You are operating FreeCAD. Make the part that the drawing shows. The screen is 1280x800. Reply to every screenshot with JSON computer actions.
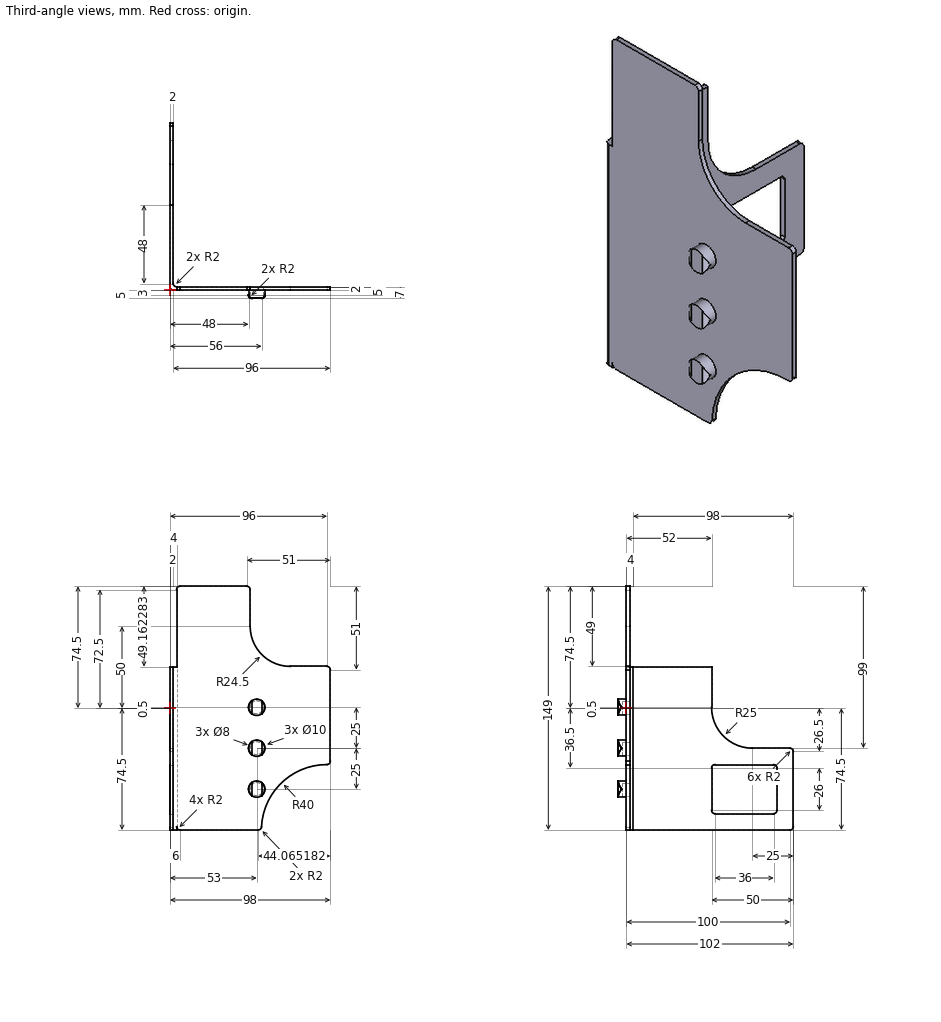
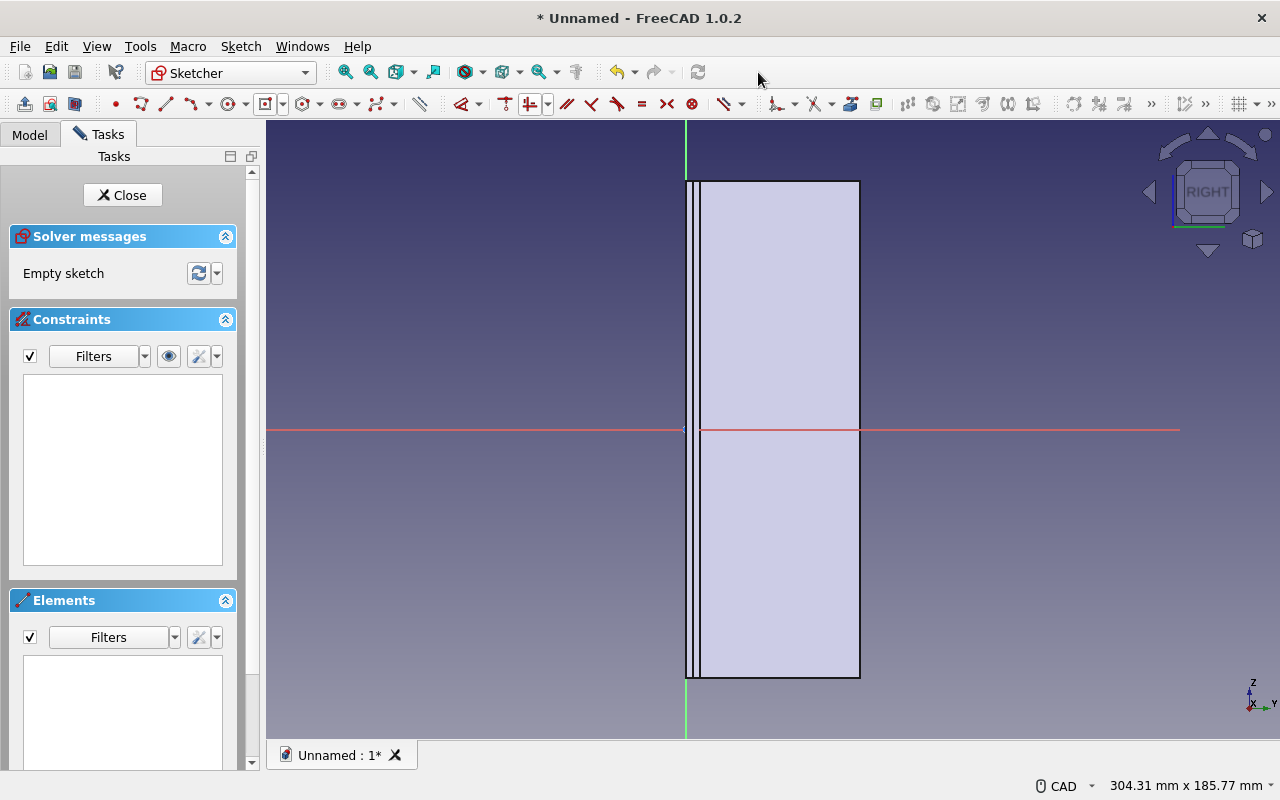
{"action": "key", "text": "q s"}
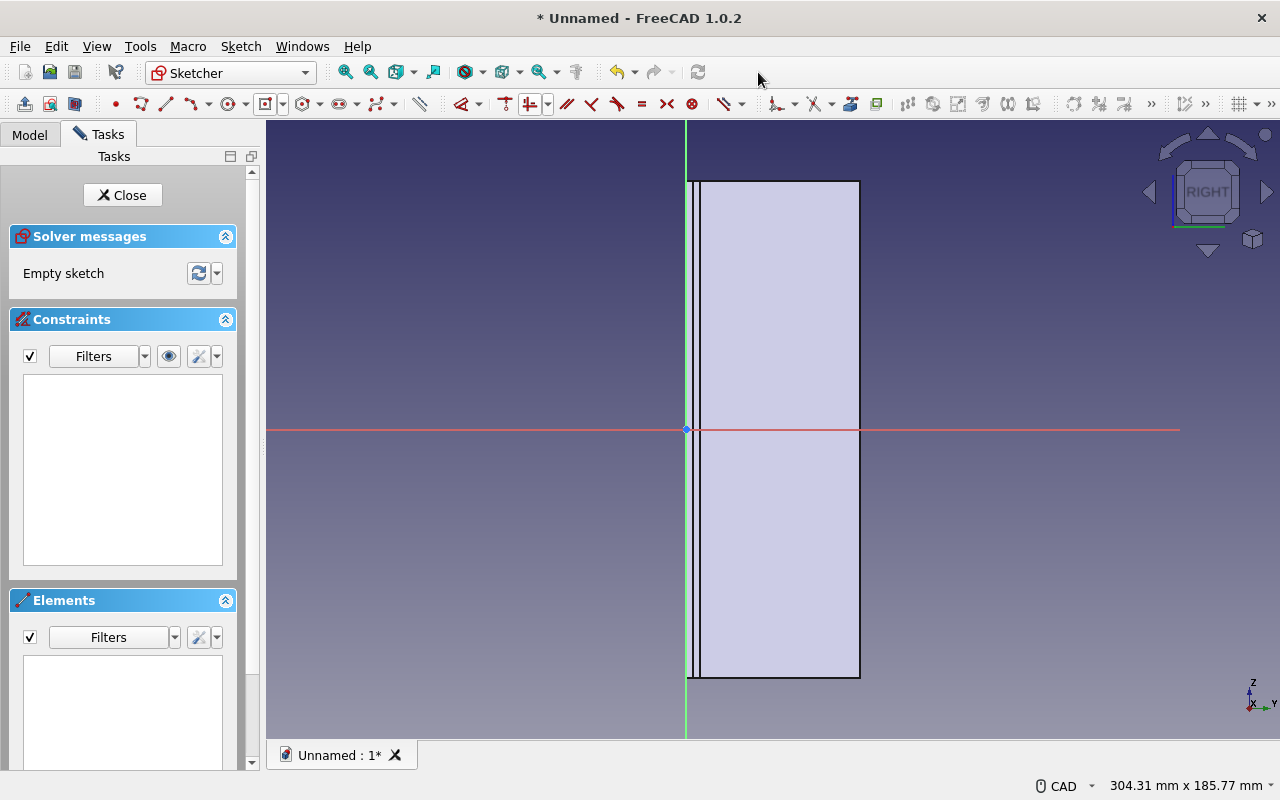
{"action": "left_click", "coordinate": [282, 104]}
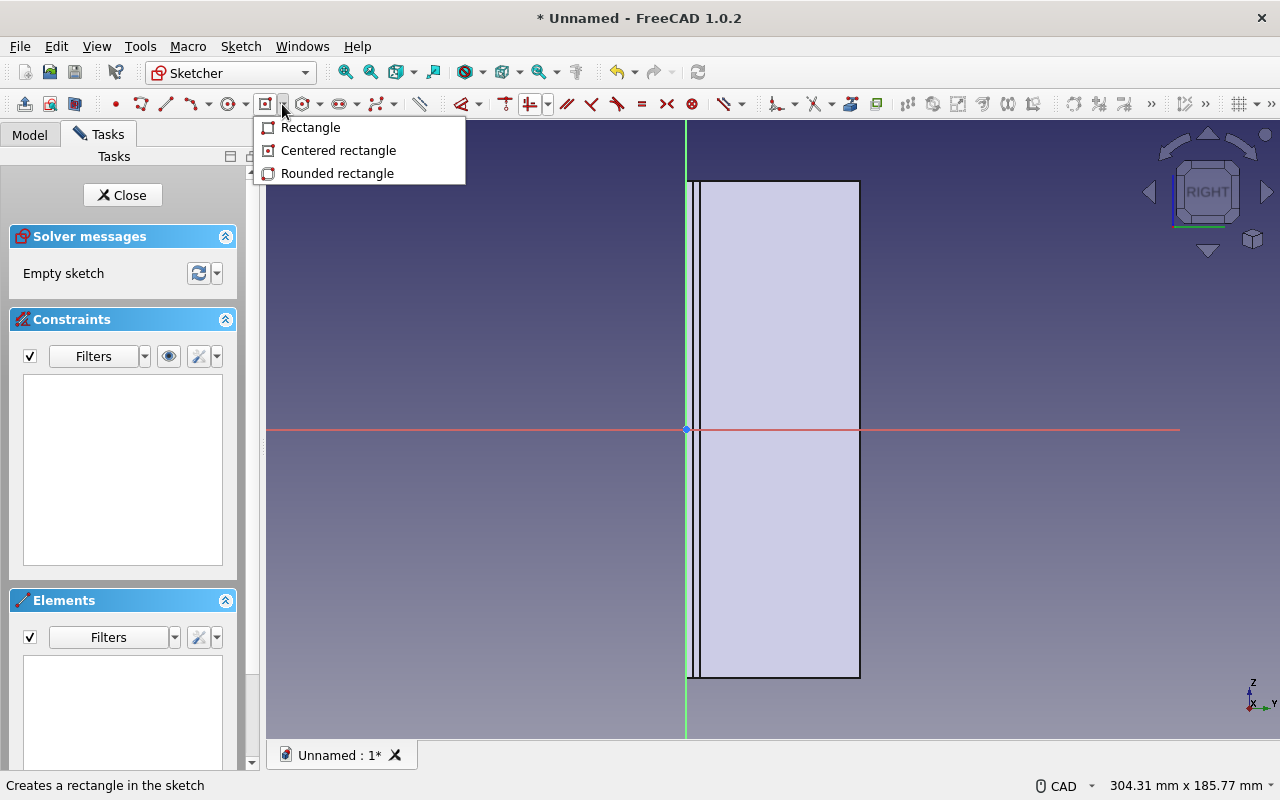
{"action": "left_click", "coordinate": [360, 128]}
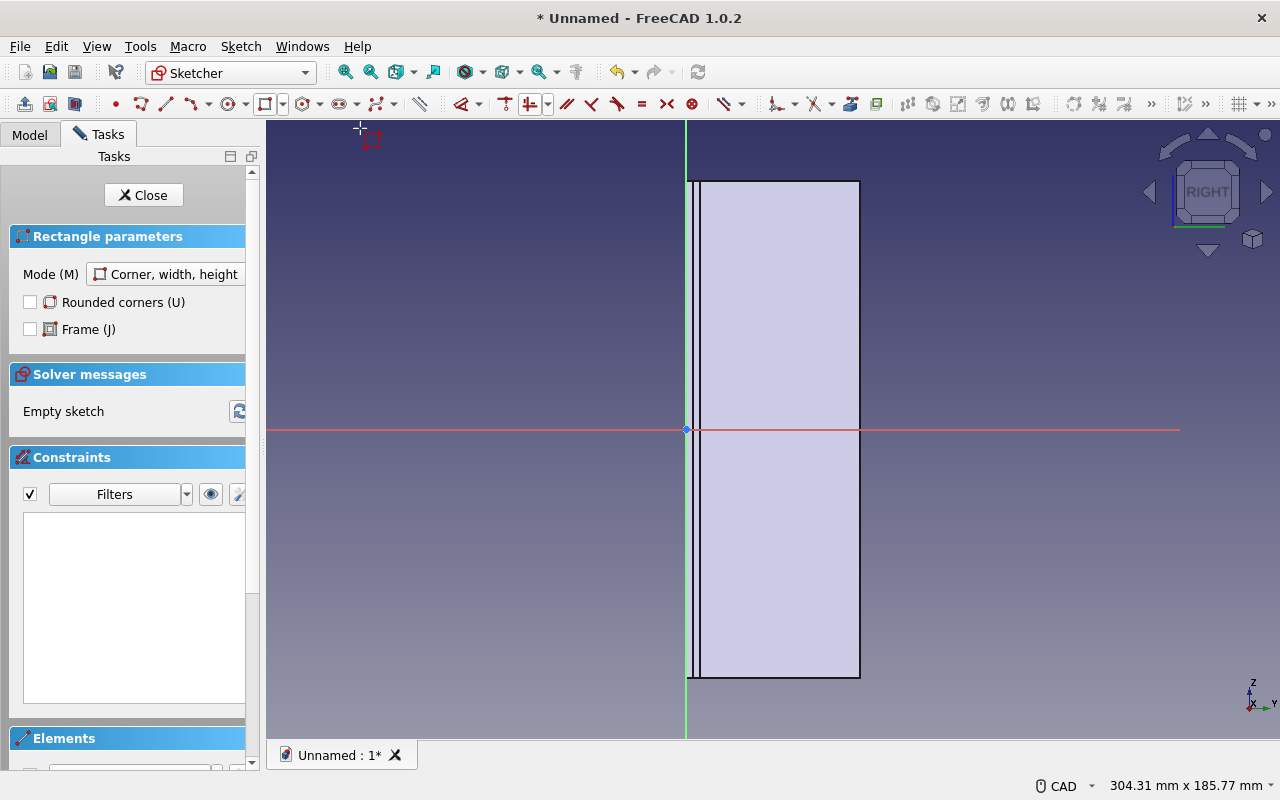
{"action": "left_click", "coordinate": [860, 181]}
{"action": "mouse_move", "coordinate": [1026, 678]}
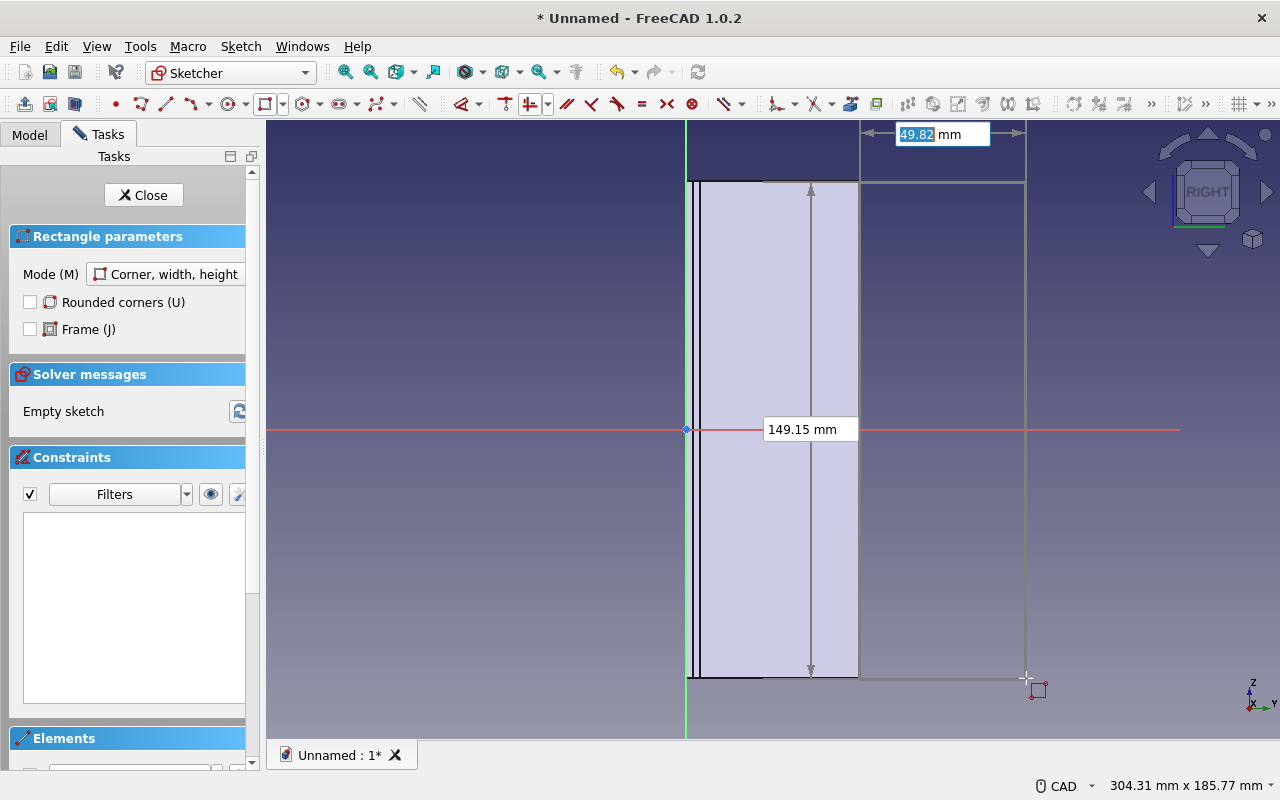
{"action": "type", "text": "50"}
{"action": "key", "text": "Tab"}
{"action": "type", "text": "149"}
{"action": "key", "text": "Return"}
{"action": "key", "text": "Escape"}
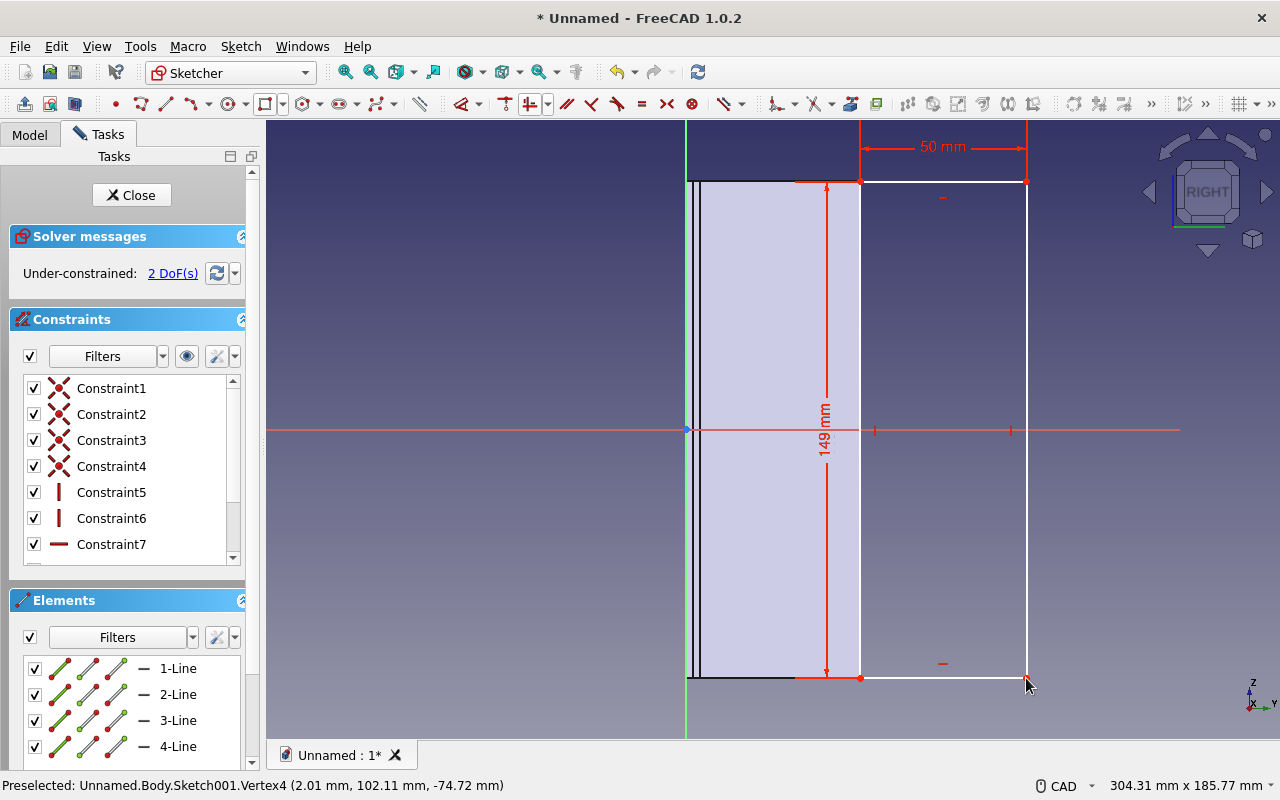
{"action": "left_click", "coordinate": [860, 182]}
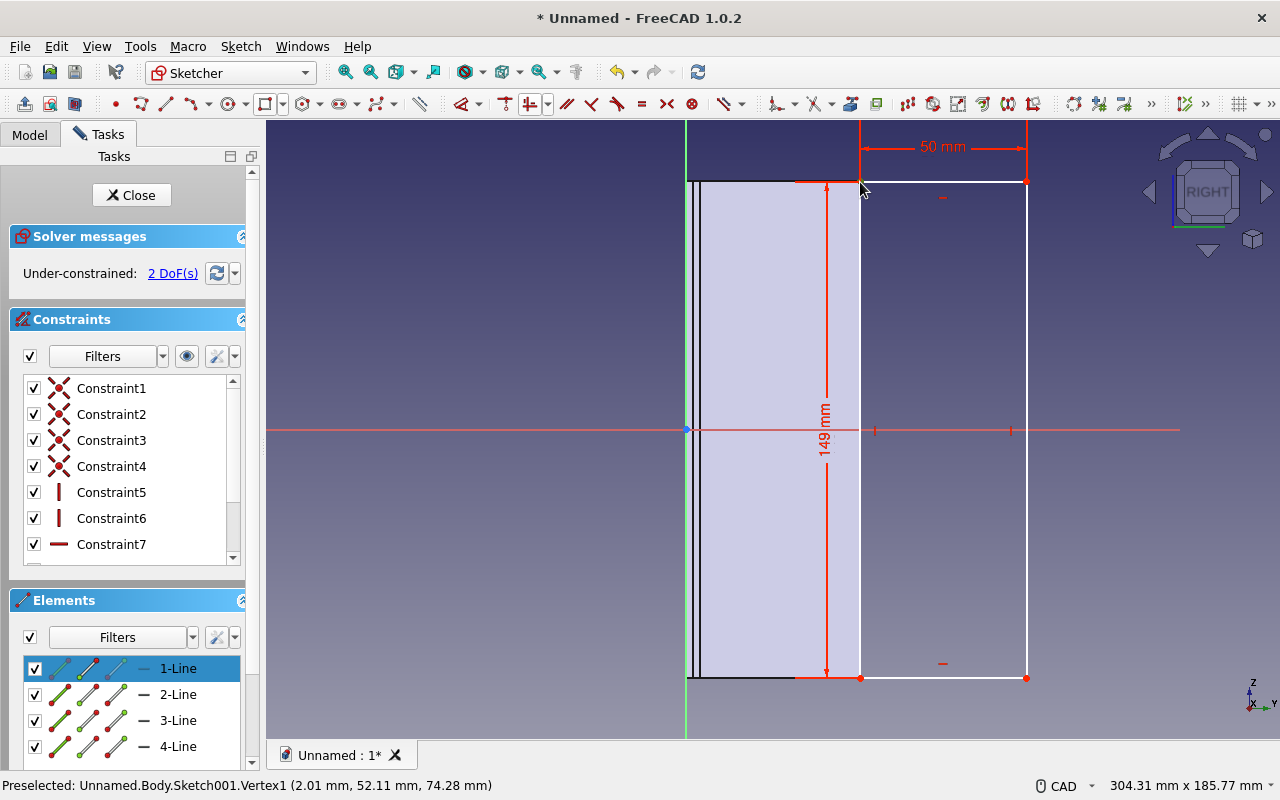
{"action": "key", "text": "l"}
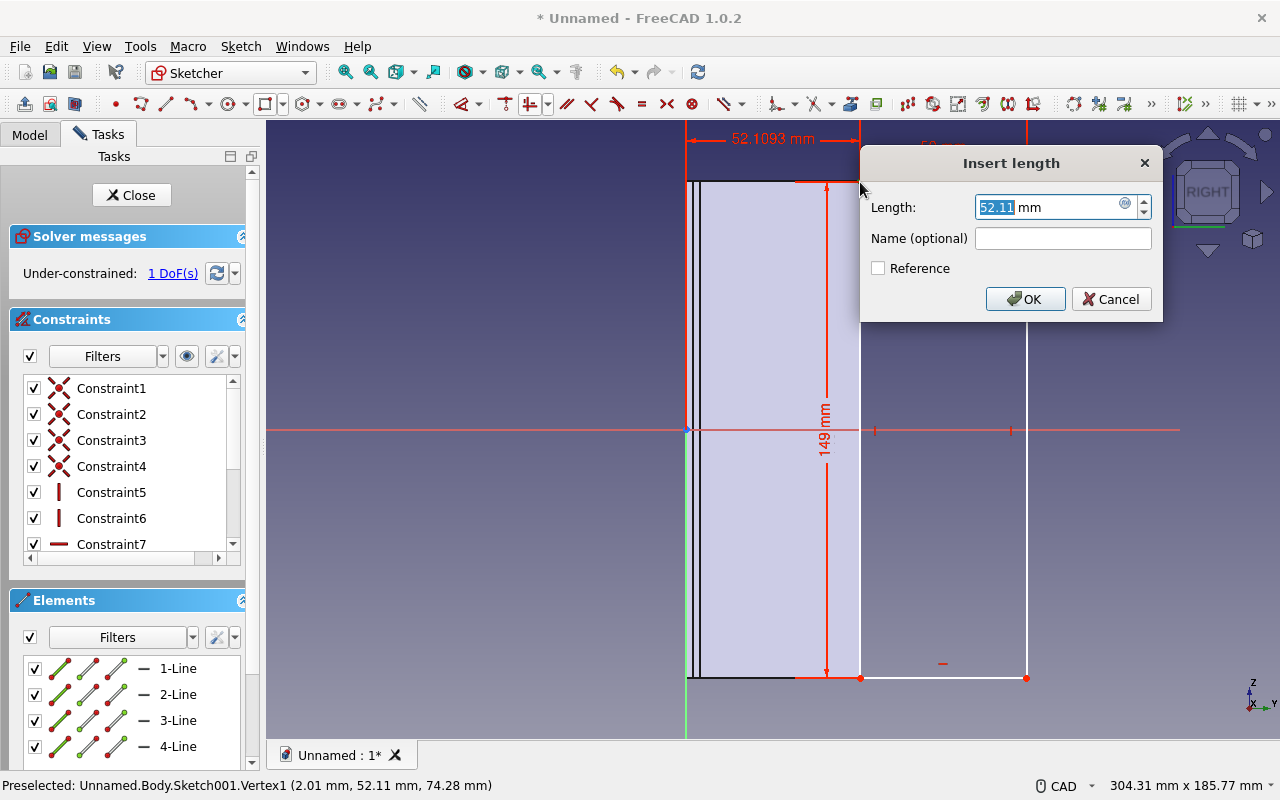
{"action": "type", "text": "52"}
{"action": "key", "text": "Return"}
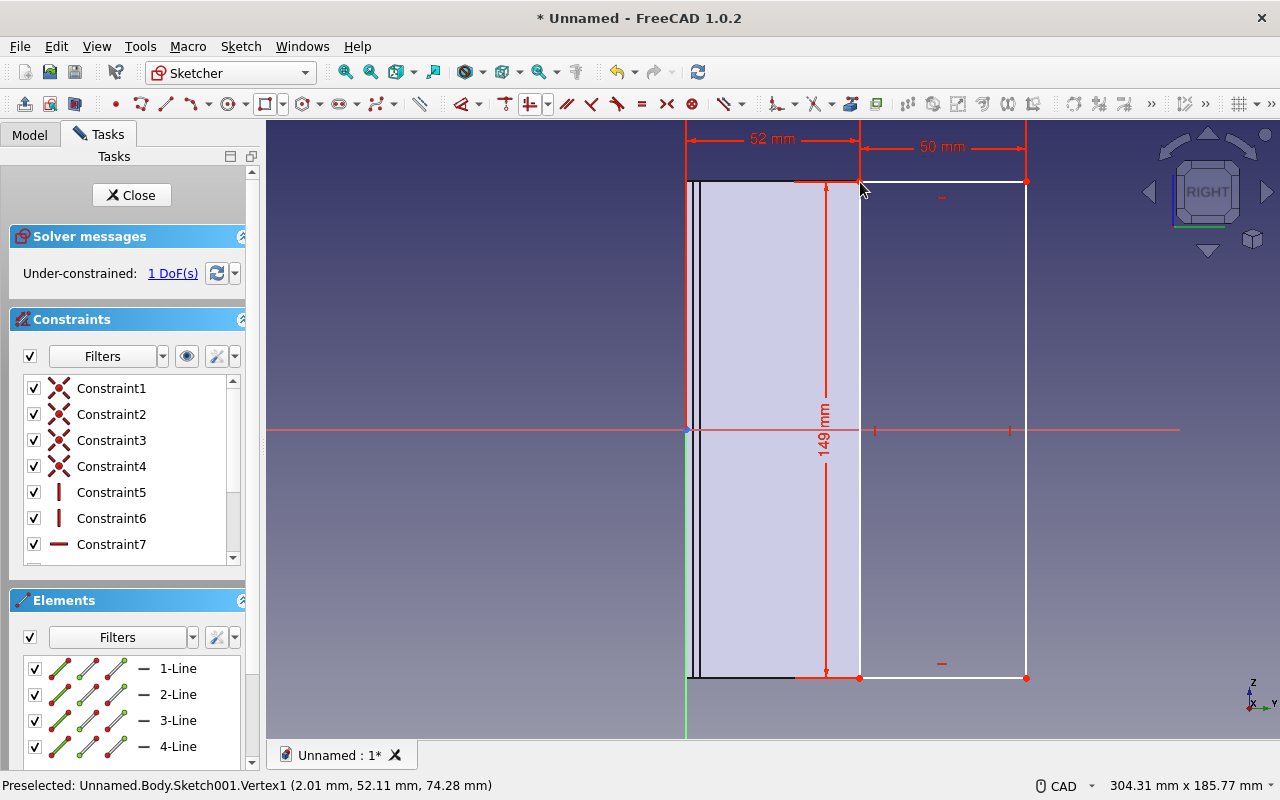
{"action": "left_click", "coordinate": [860, 182]}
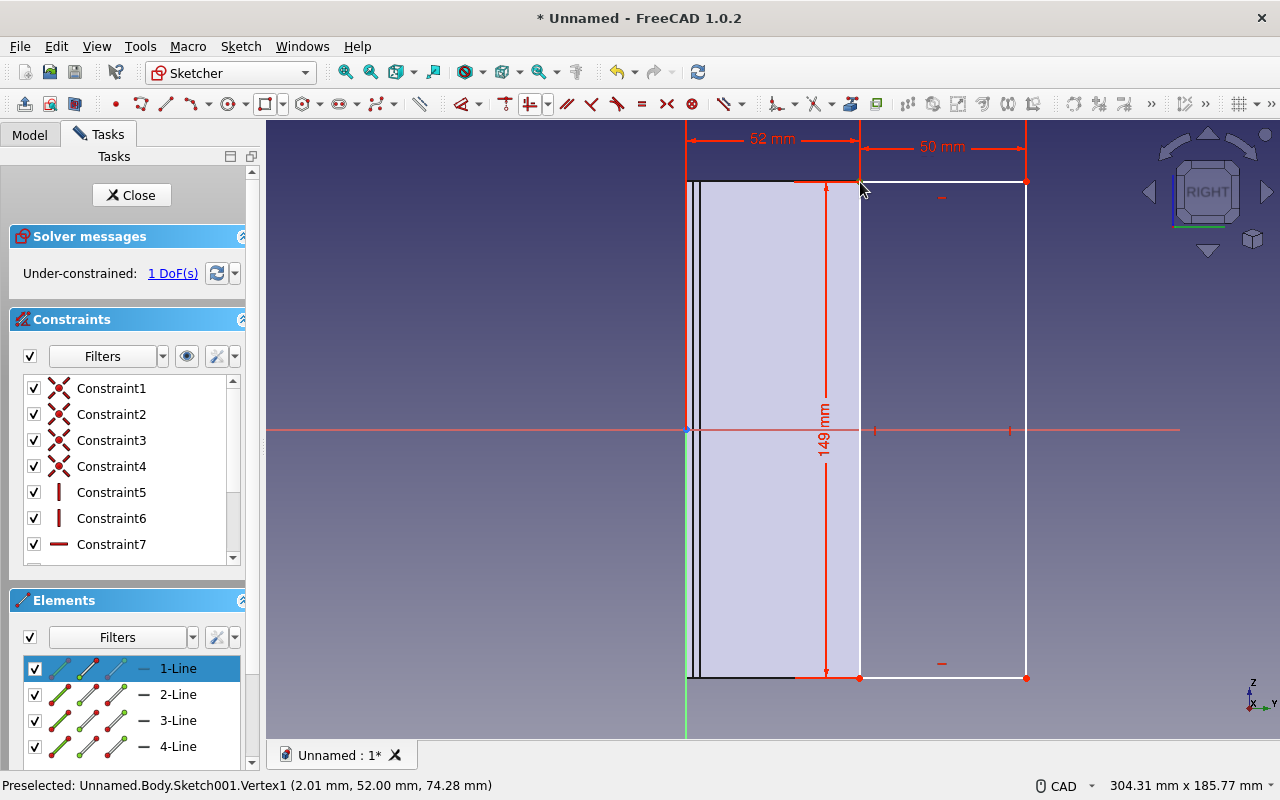
{"action": "key", "text": "i"}